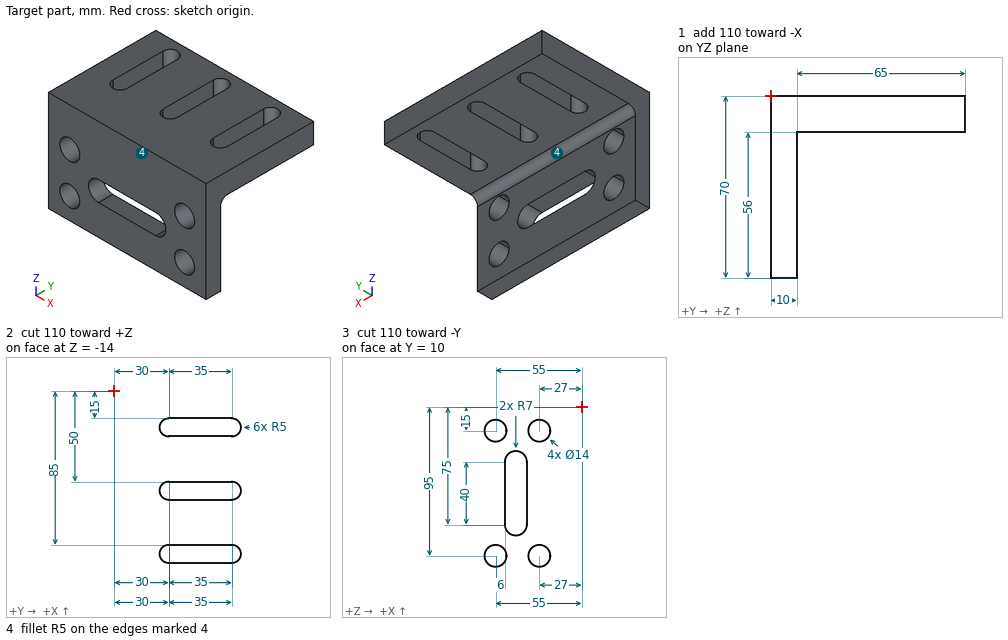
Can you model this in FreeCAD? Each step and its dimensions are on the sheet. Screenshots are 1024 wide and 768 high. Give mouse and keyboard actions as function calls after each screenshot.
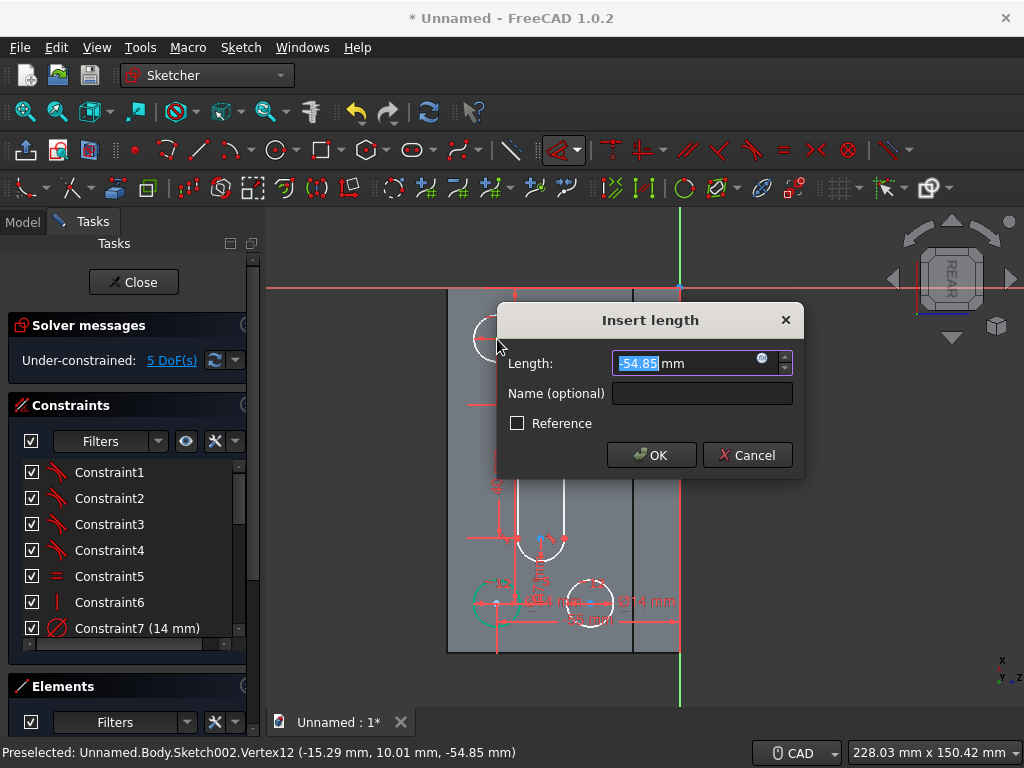
text(-55)
key(Return)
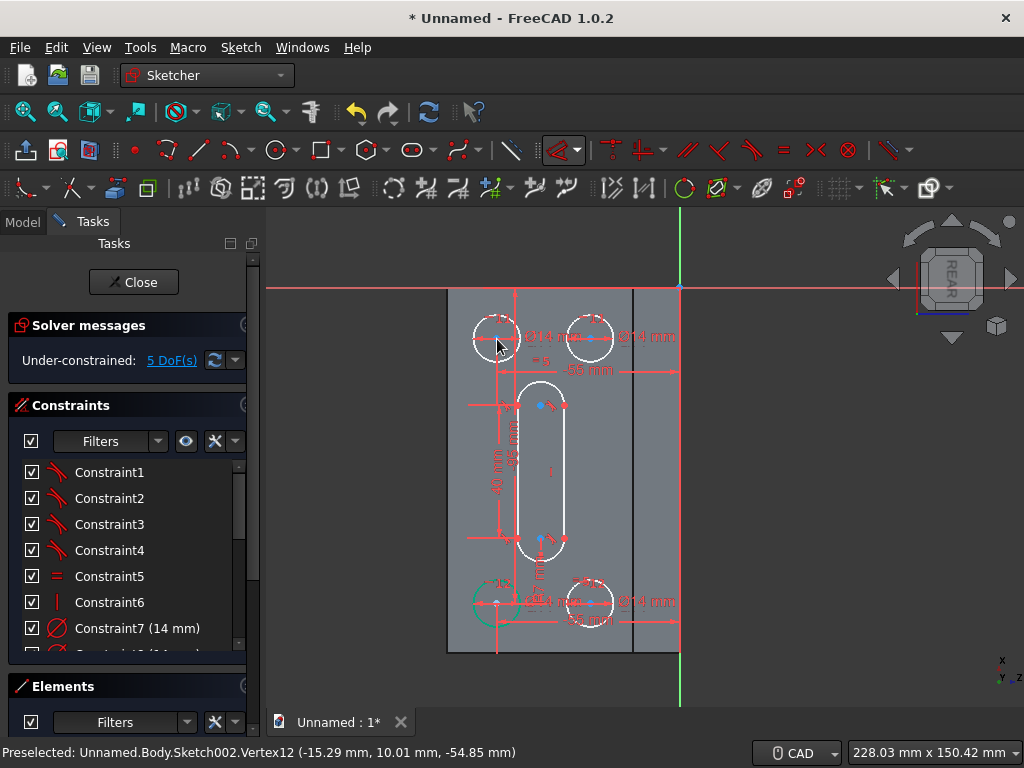
click(497, 339)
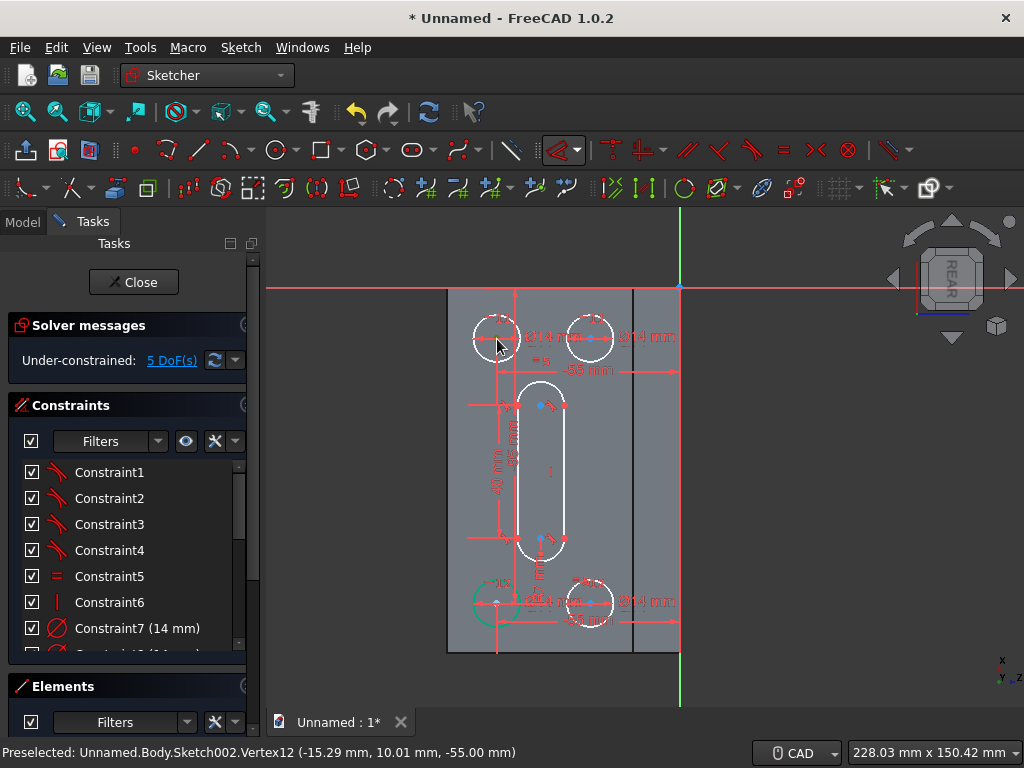
click(580, 150)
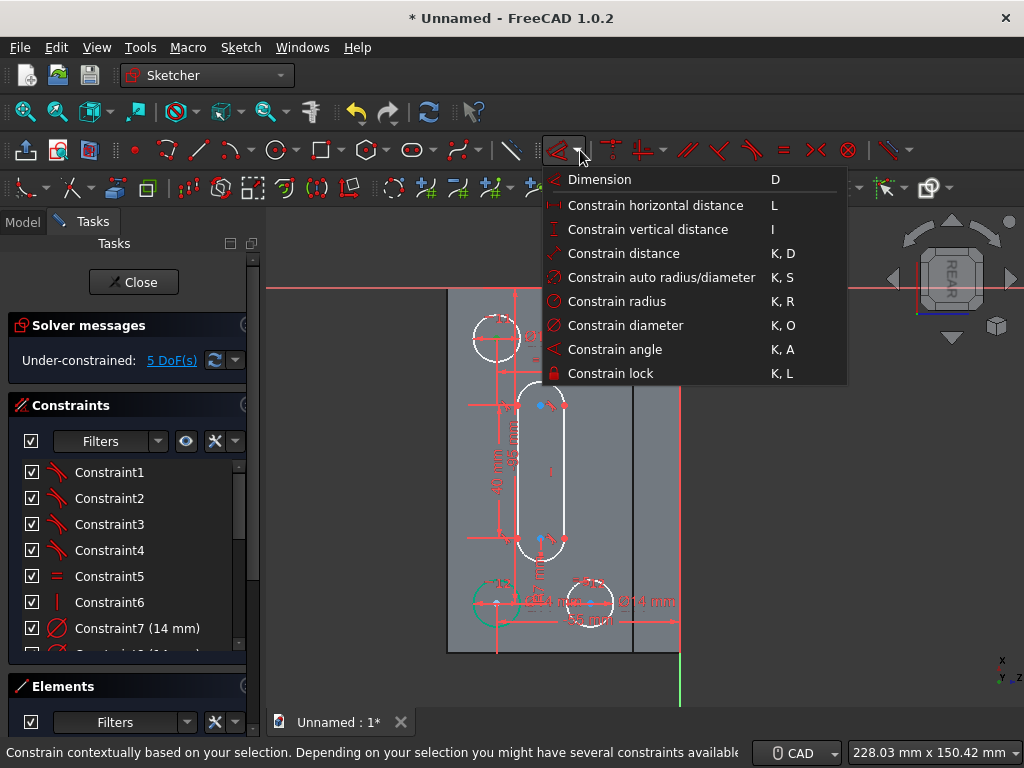
click(695, 229)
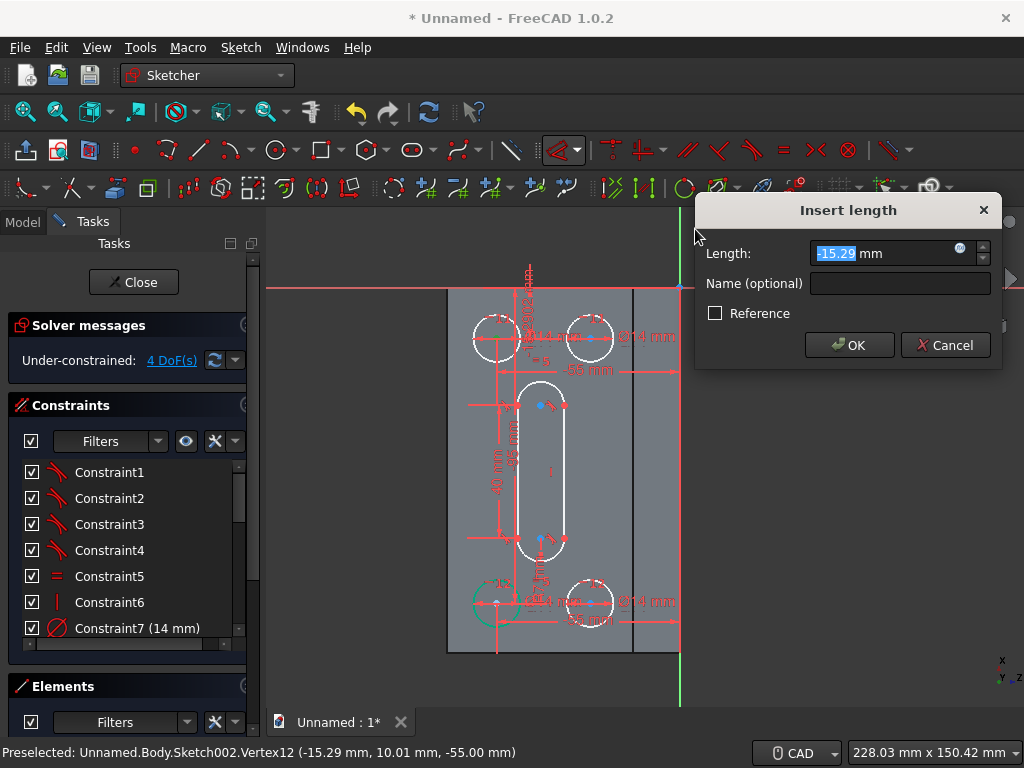
text(-15)
key(Return)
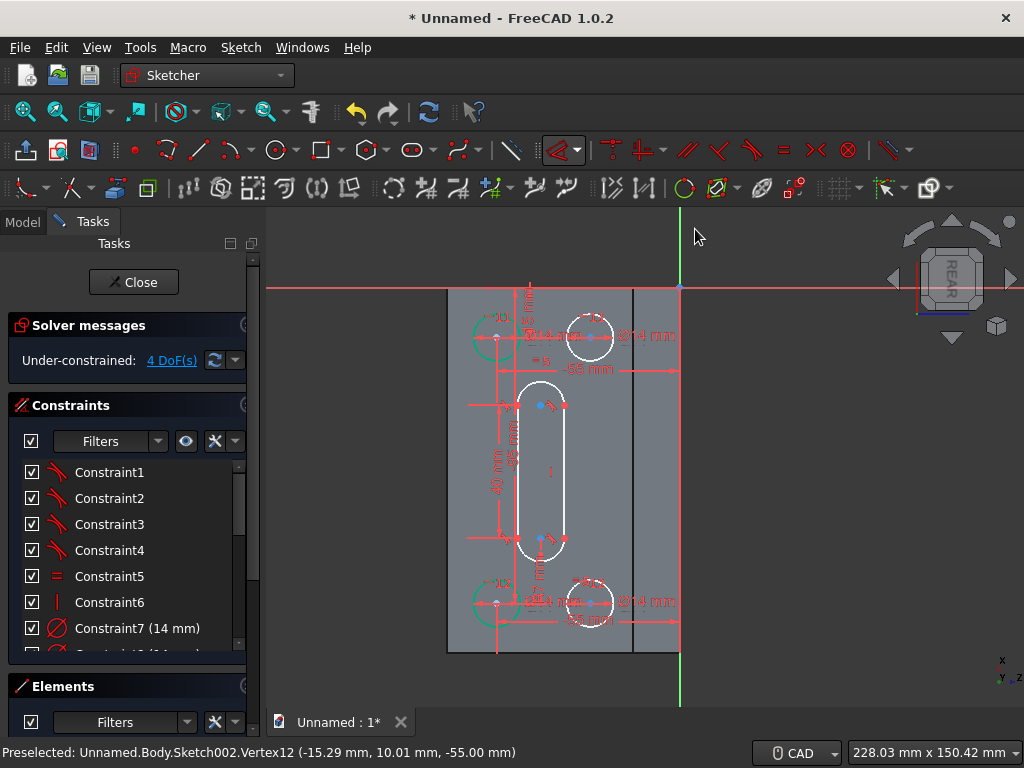
click(590, 338)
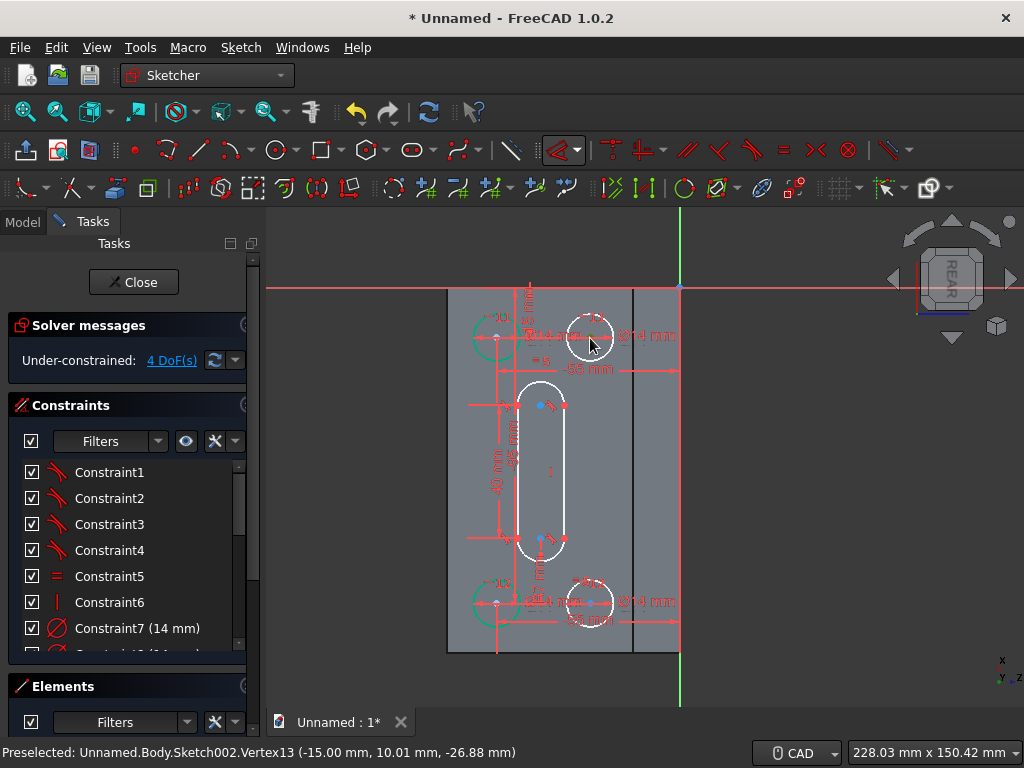
key(l)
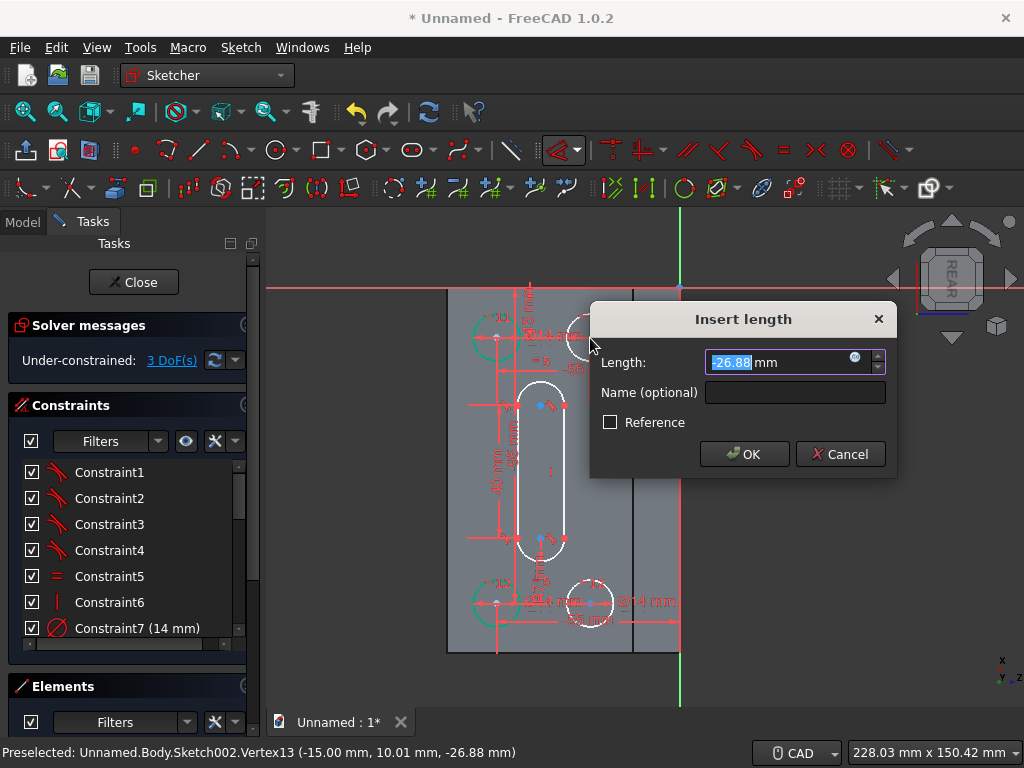
text(-27)
key(Return)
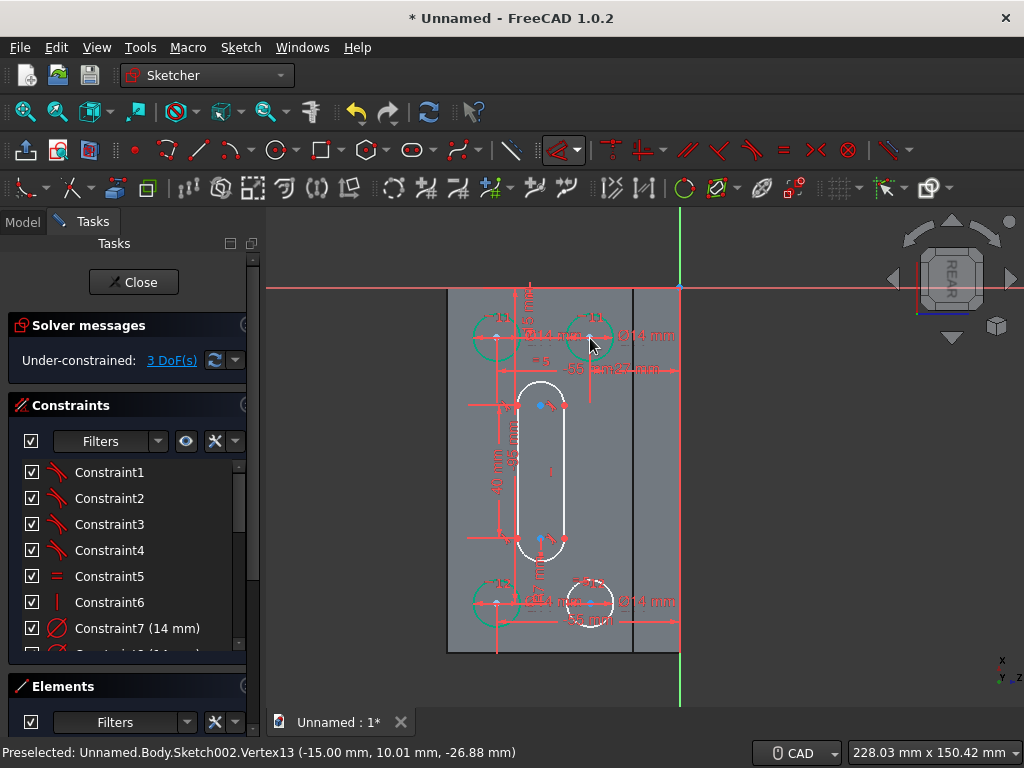
click(590, 604)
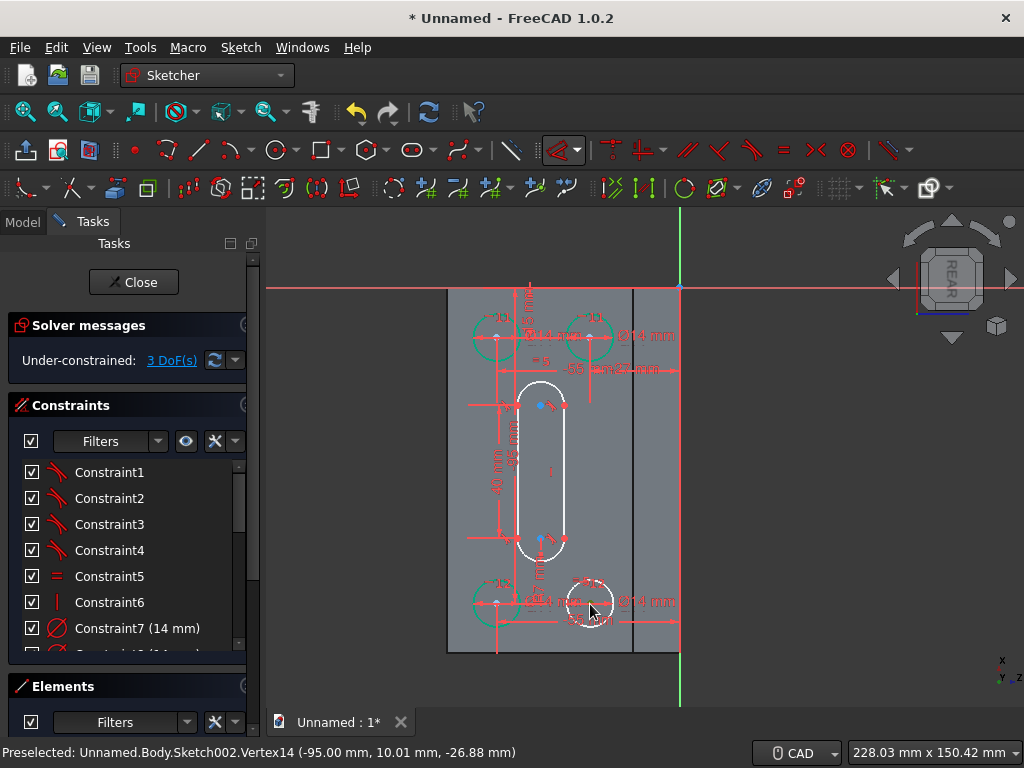
key(l)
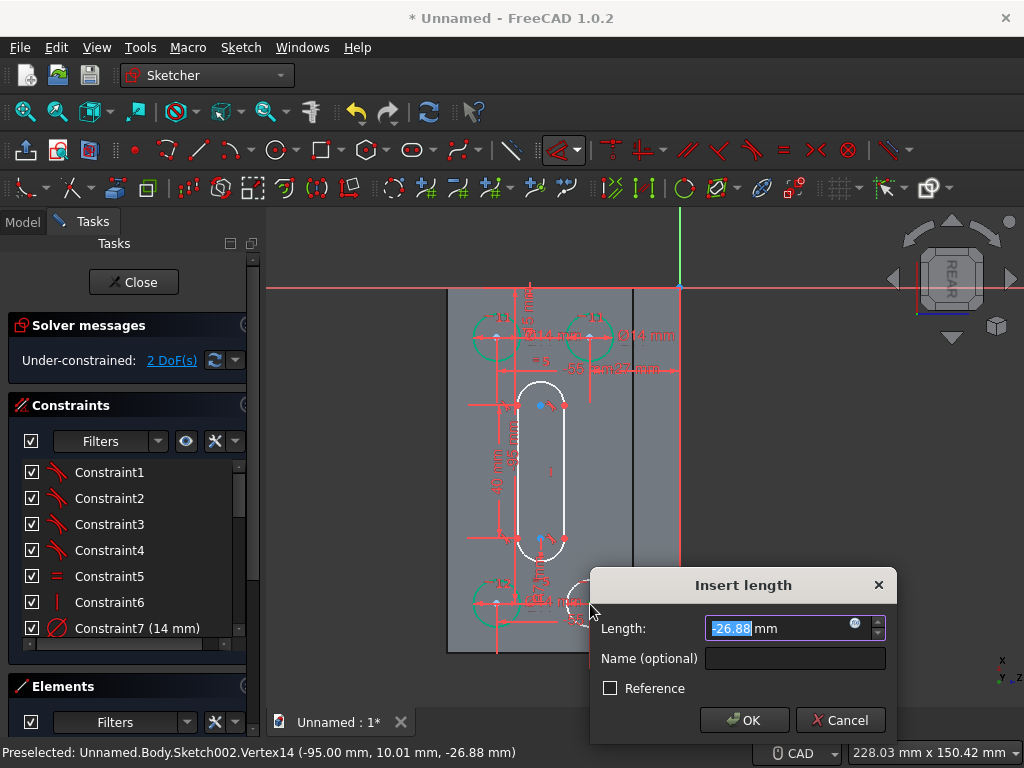
text(-27)
key(Return)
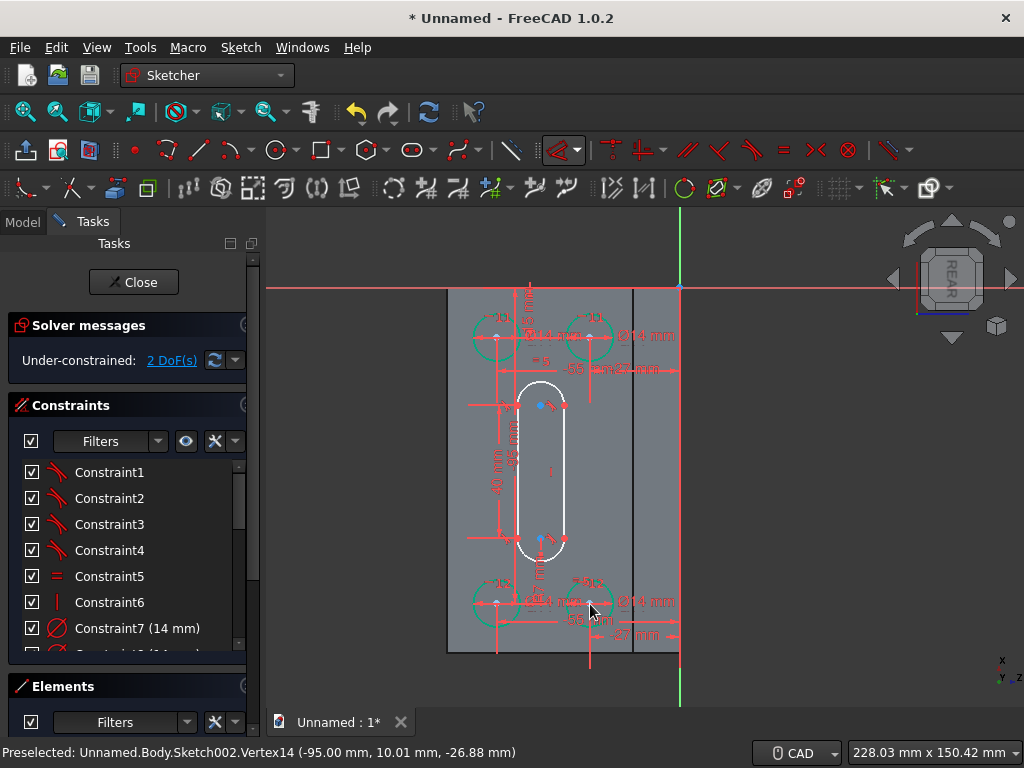
scroll(518, 538, up, 4)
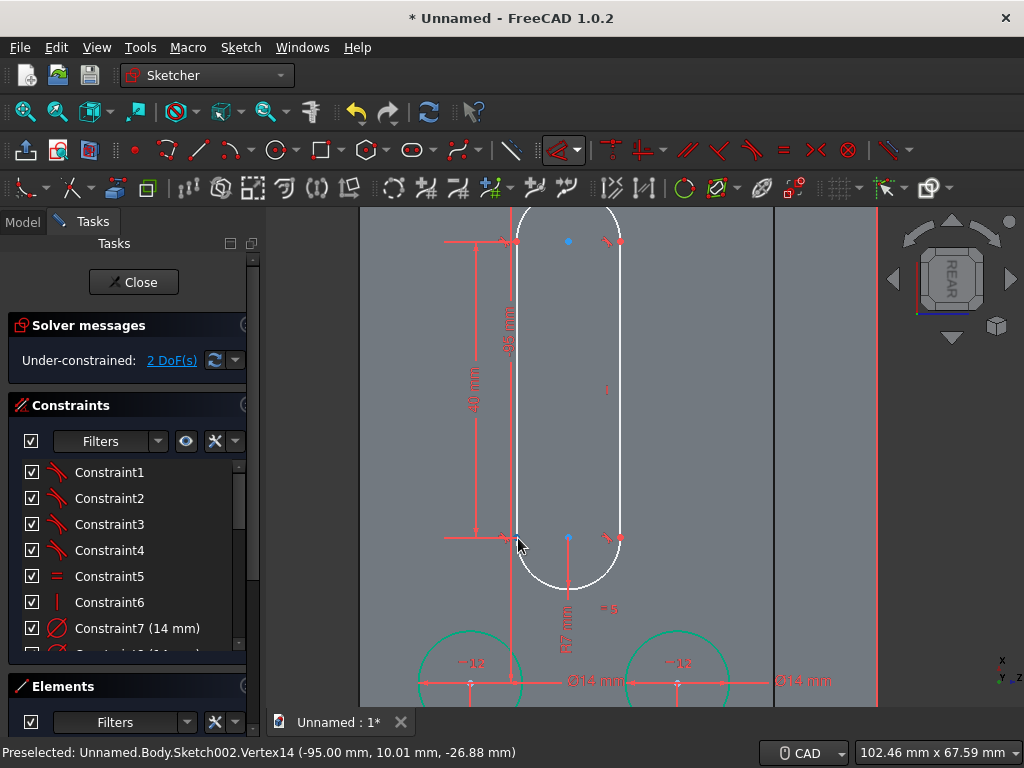
click(517, 538)